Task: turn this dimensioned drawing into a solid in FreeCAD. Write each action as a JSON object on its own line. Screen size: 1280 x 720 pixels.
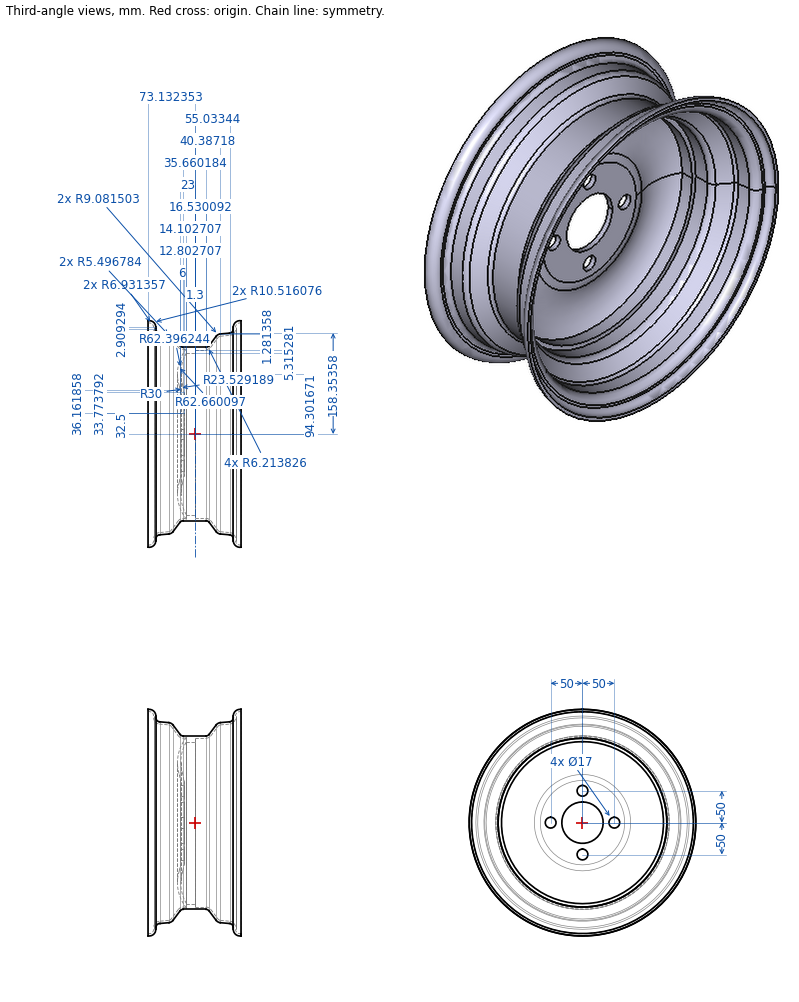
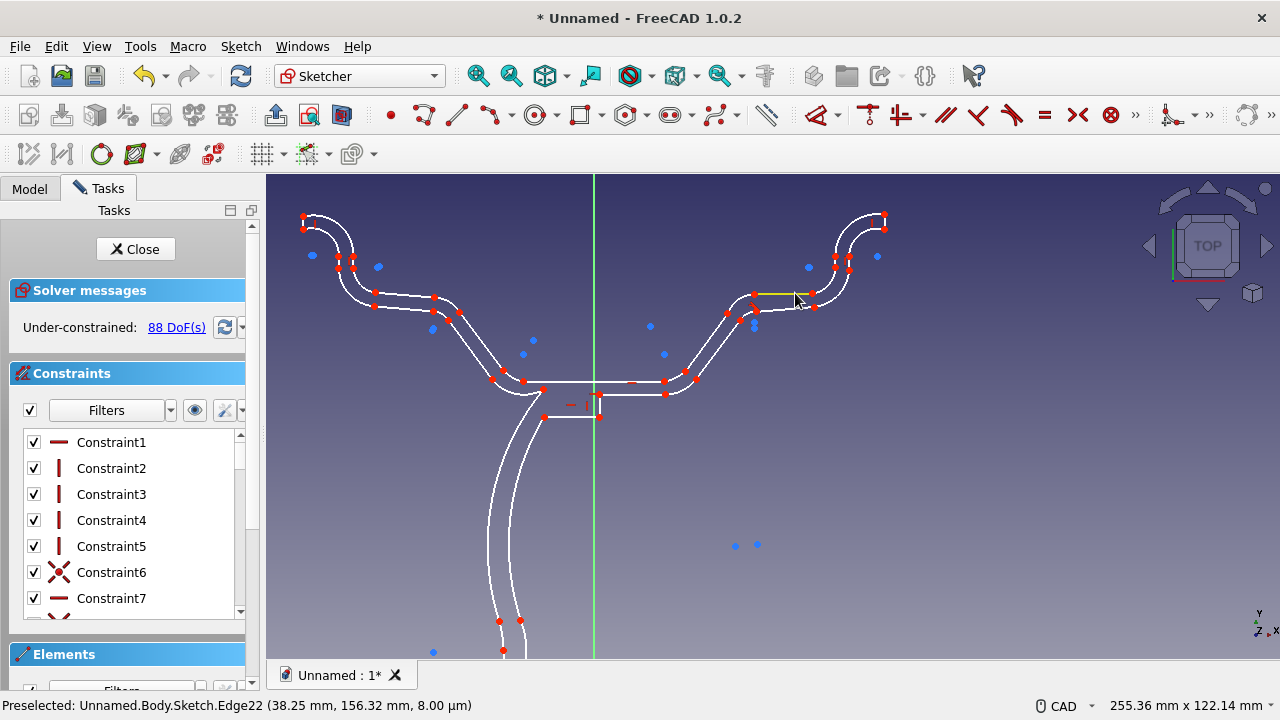
{"action": "left_click", "coordinate": [795, 294]}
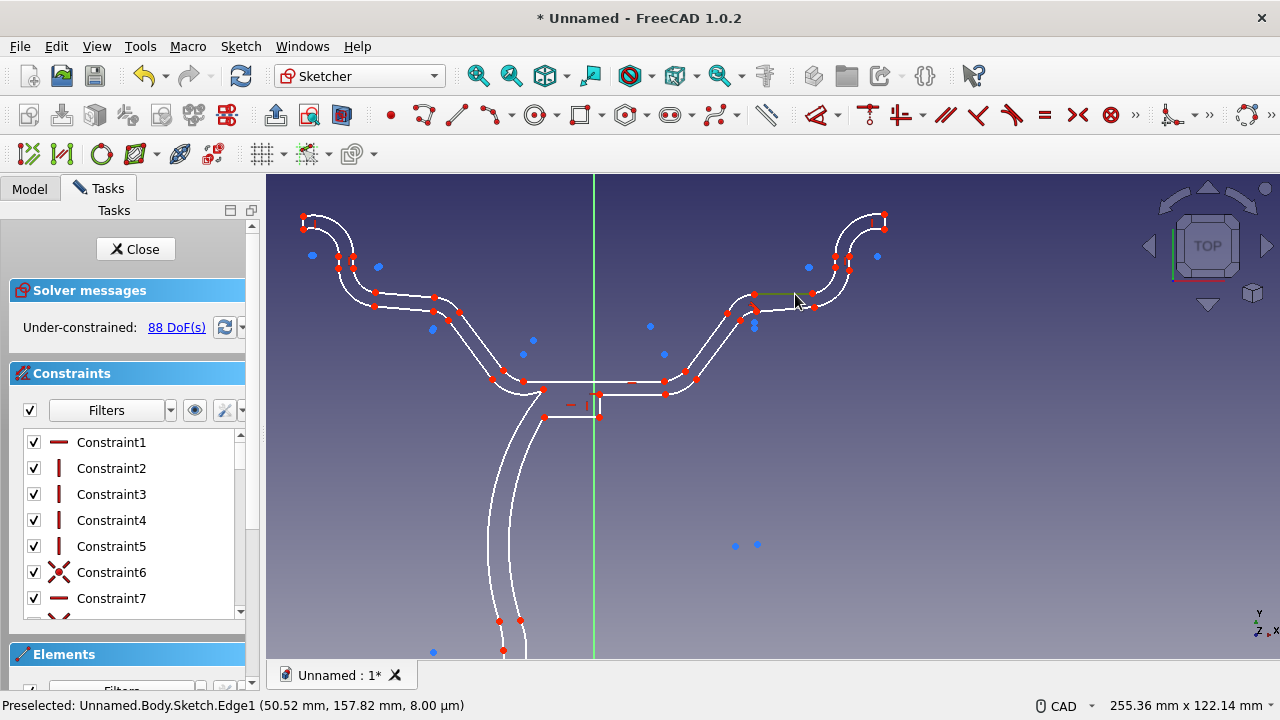
{"action": "scroll", "coordinate": [823, 290], "scroll_direction": "up", "scroll_amount": 2}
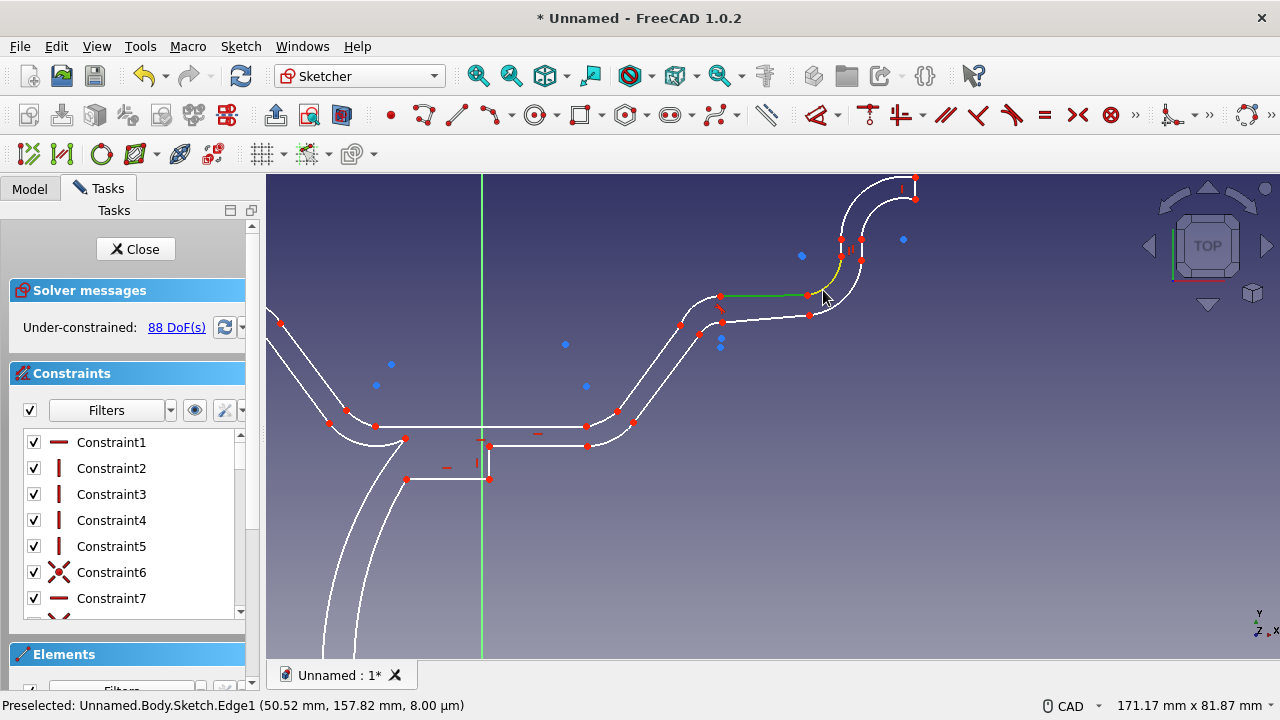
{"action": "left_click", "coordinate": [823, 289]}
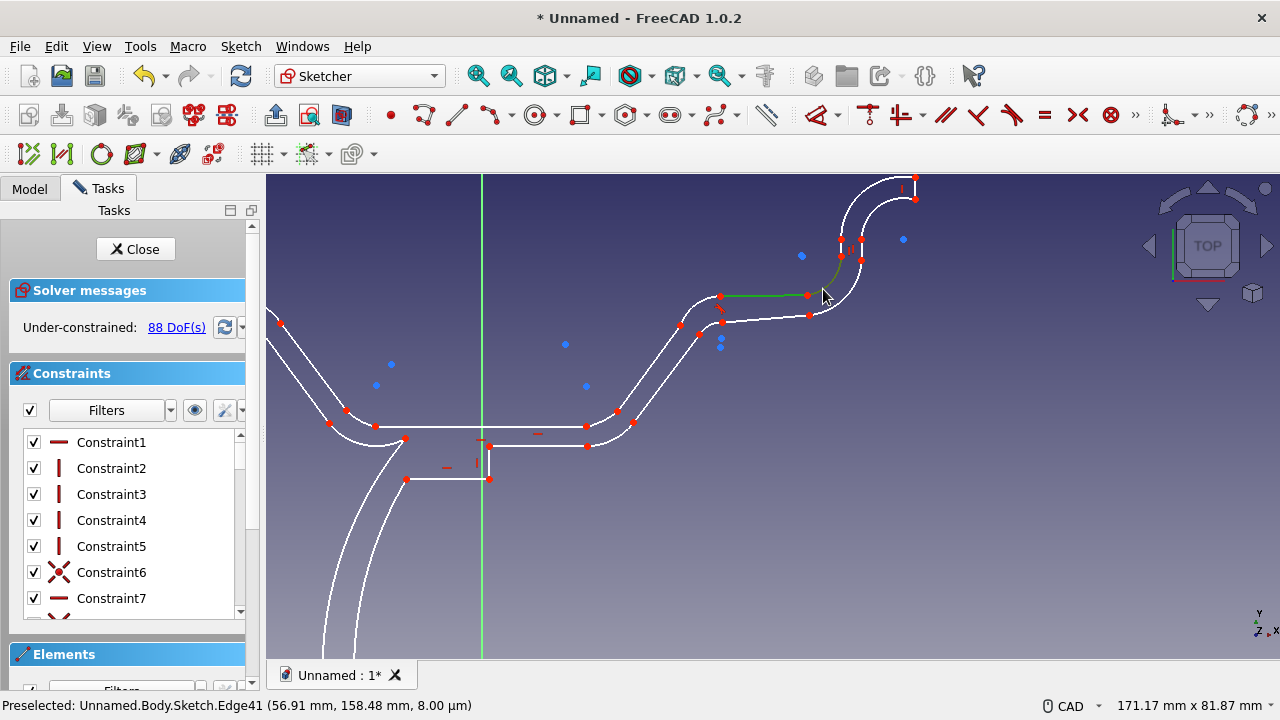
{"action": "key", "text": "t"}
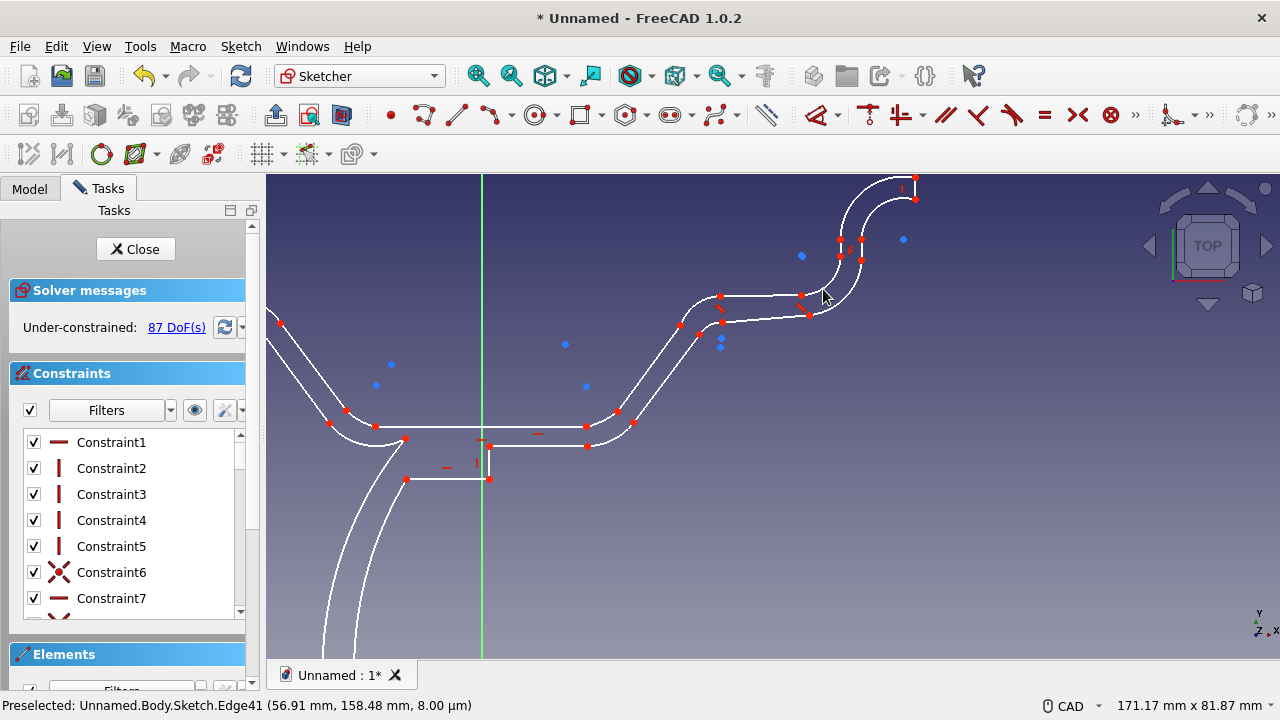
{"action": "left_click", "coordinate": [662, 351]}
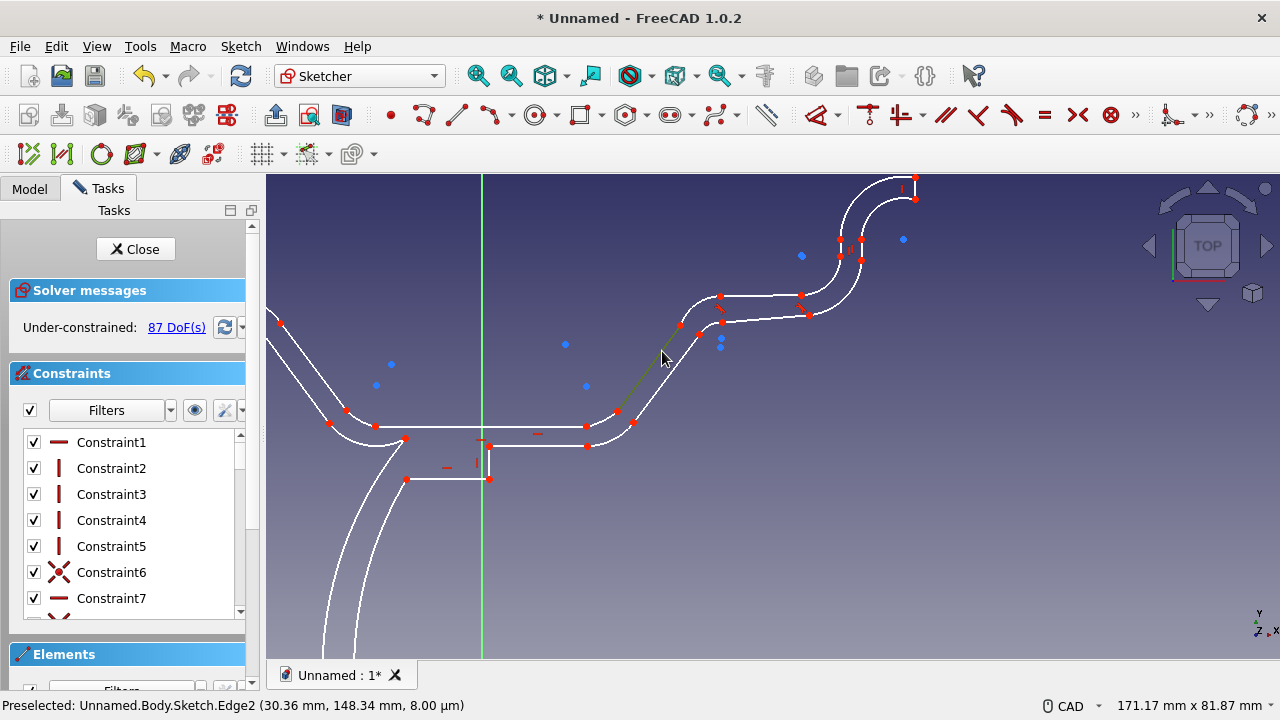
{"action": "left_click", "coordinate": [705, 299]}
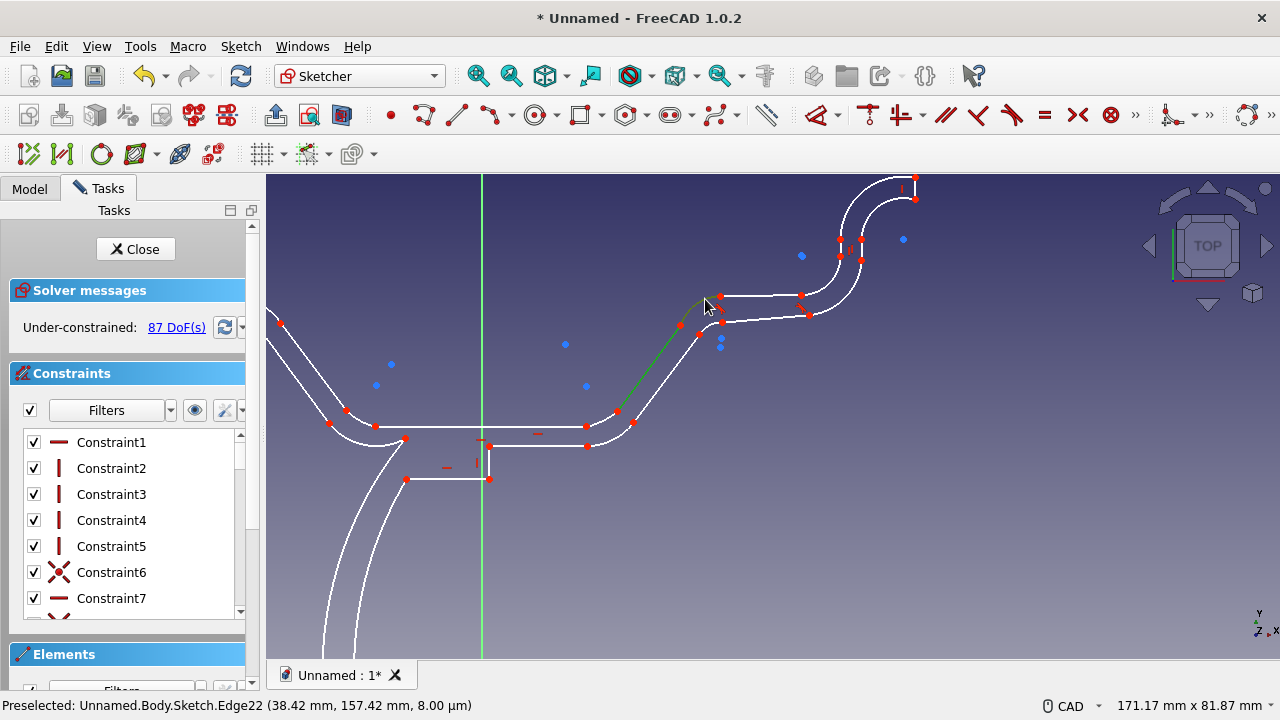
{"action": "left_click", "coordinate": [1012, 116]}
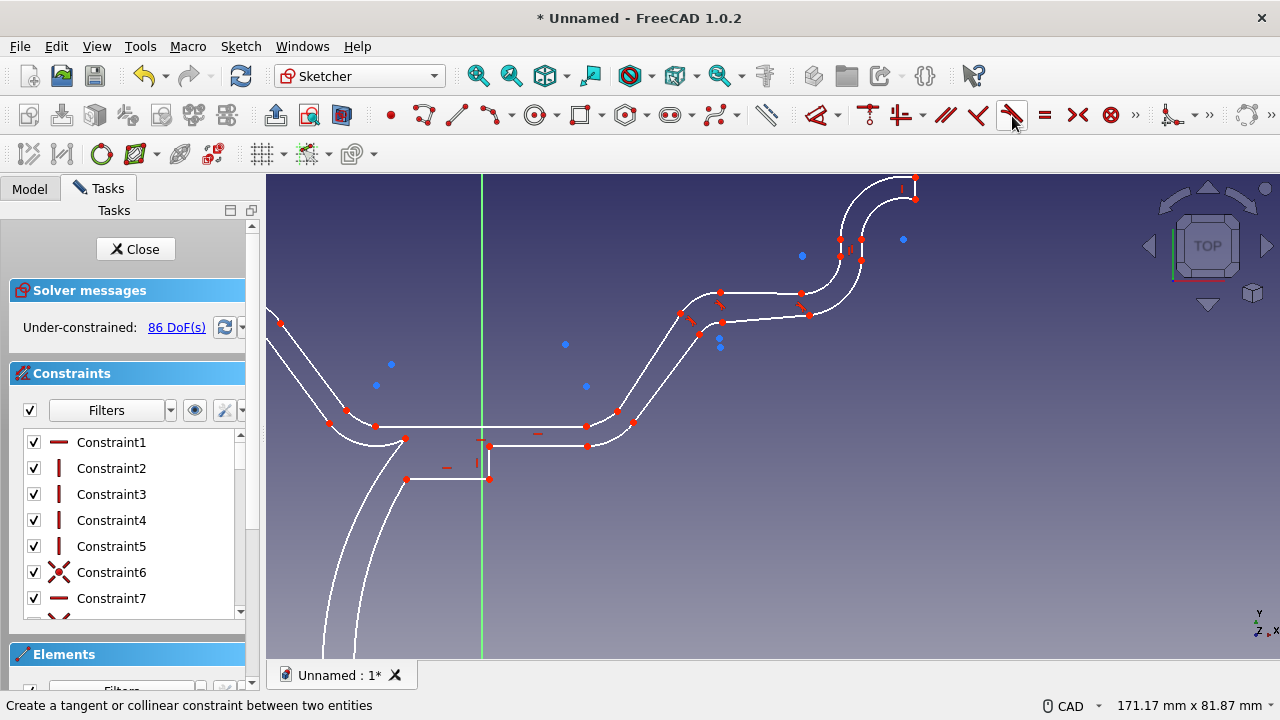
{"action": "left_click", "coordinate": [662, 343]}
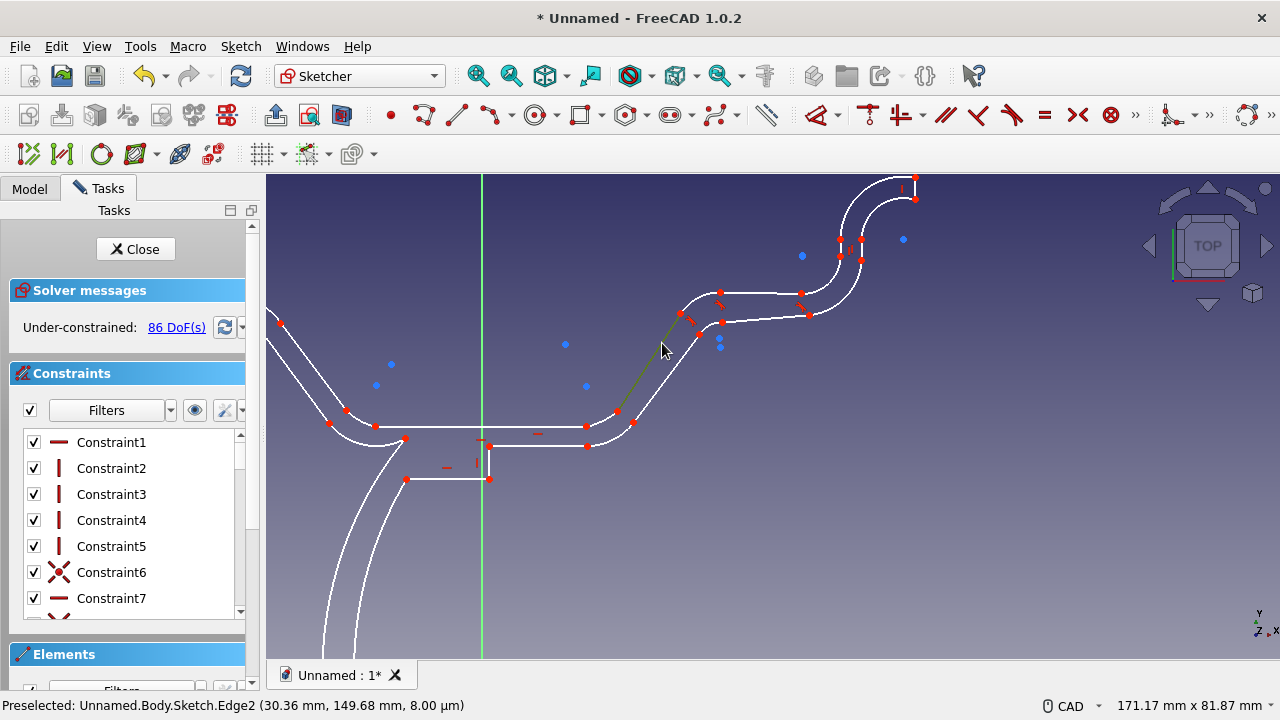
{"action": "scroll", "coordinate": [597, 424], "scroll_direction": "up", "scroll_amount": 2}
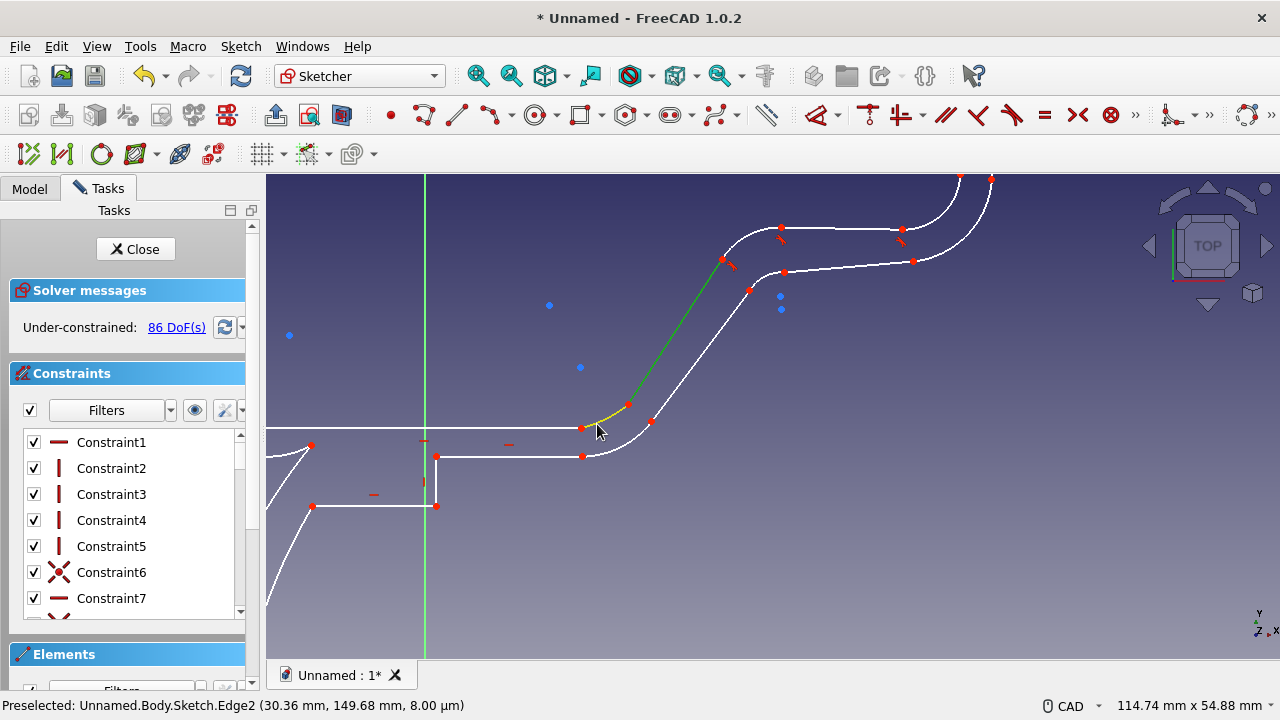
{"action": "left_click", "coordinate": [597, 423]}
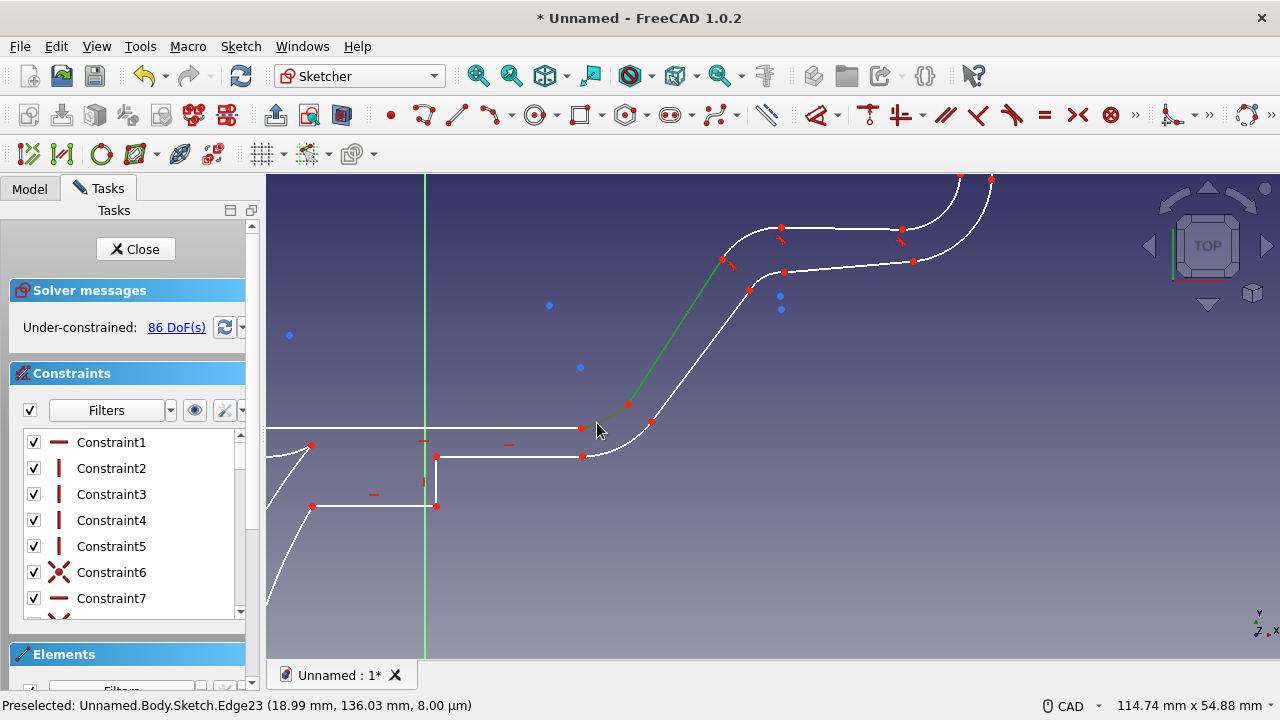
{"action": "key", "text": "t"}